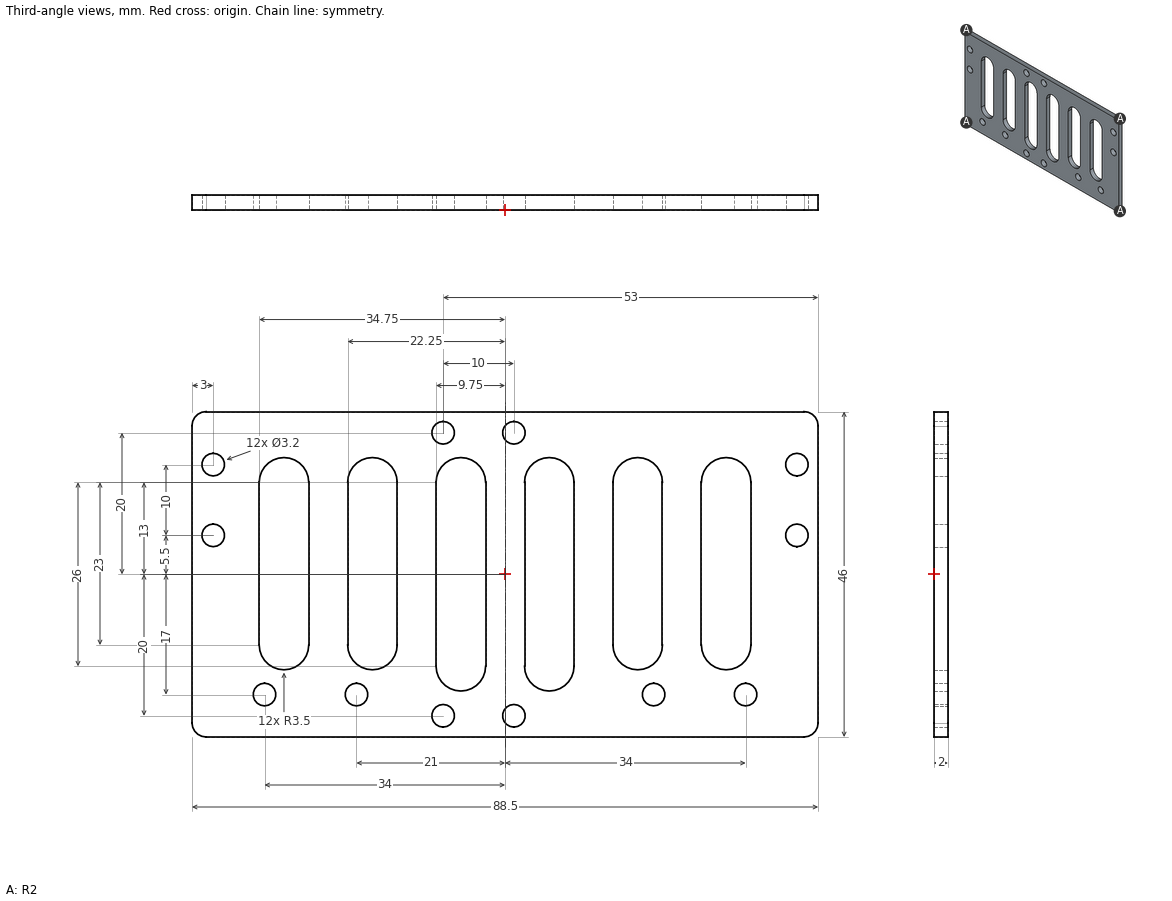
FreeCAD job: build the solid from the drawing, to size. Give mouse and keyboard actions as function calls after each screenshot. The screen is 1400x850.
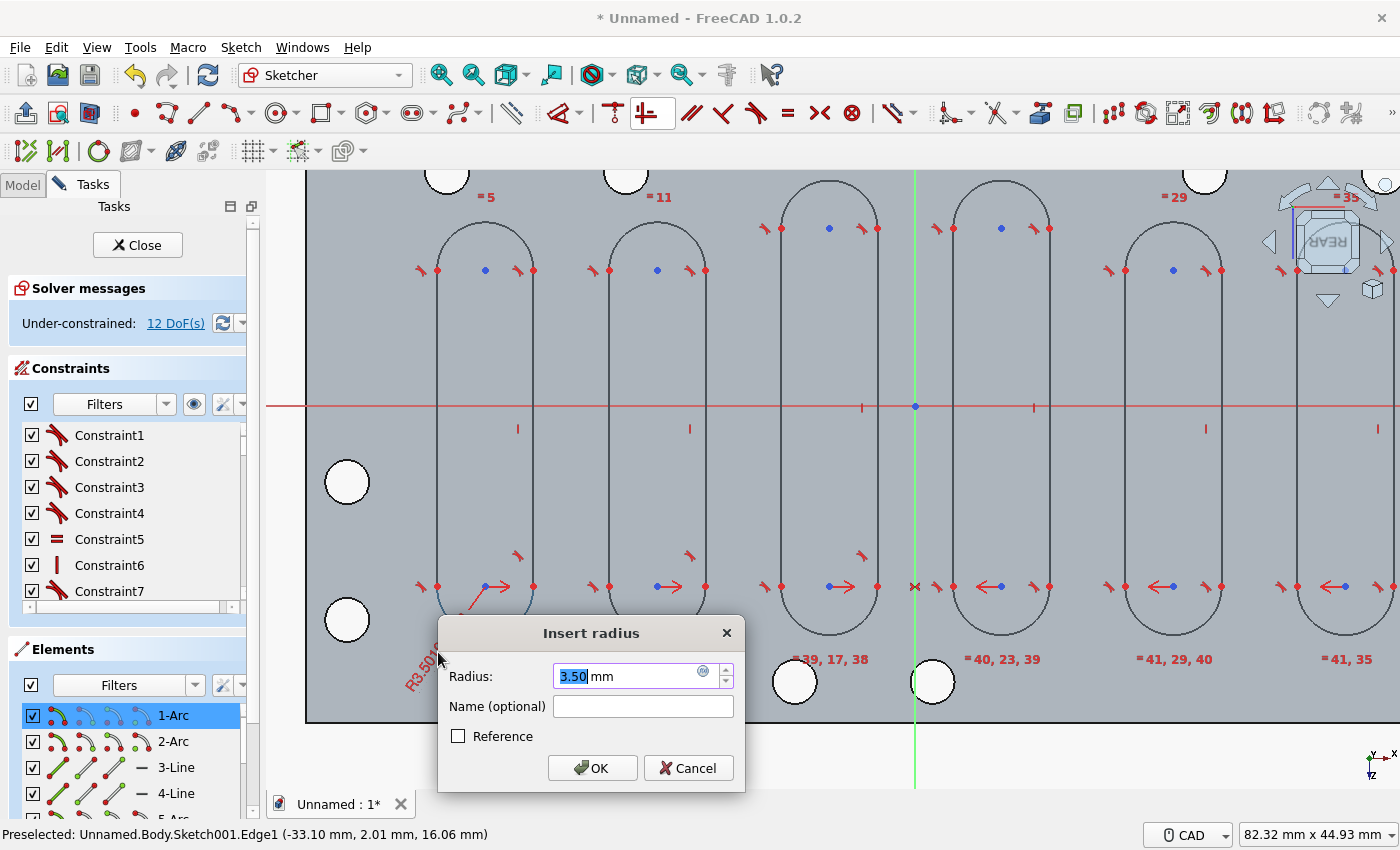
text(3.5)
key(Return)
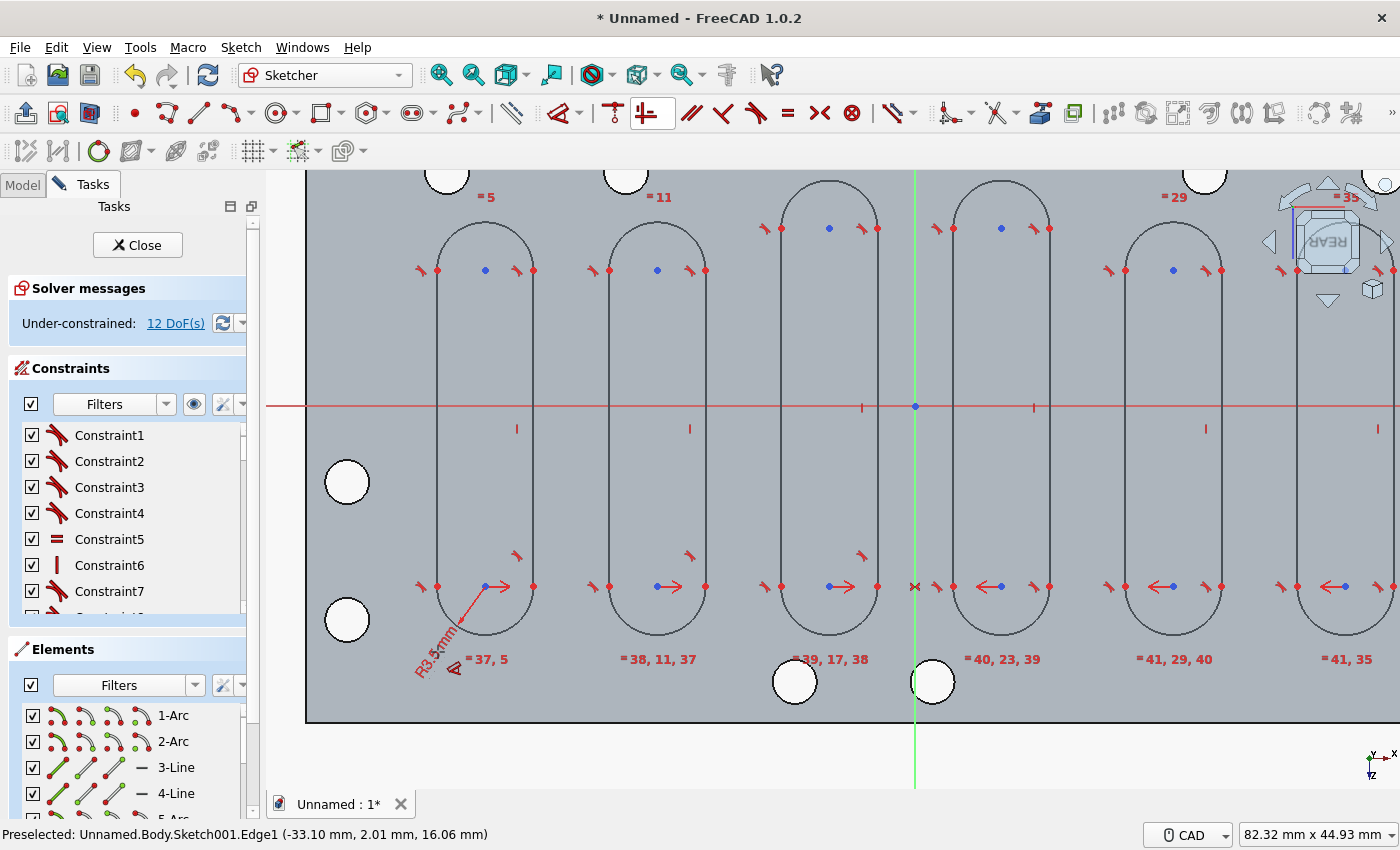
click(437, 492)
click(403, 429)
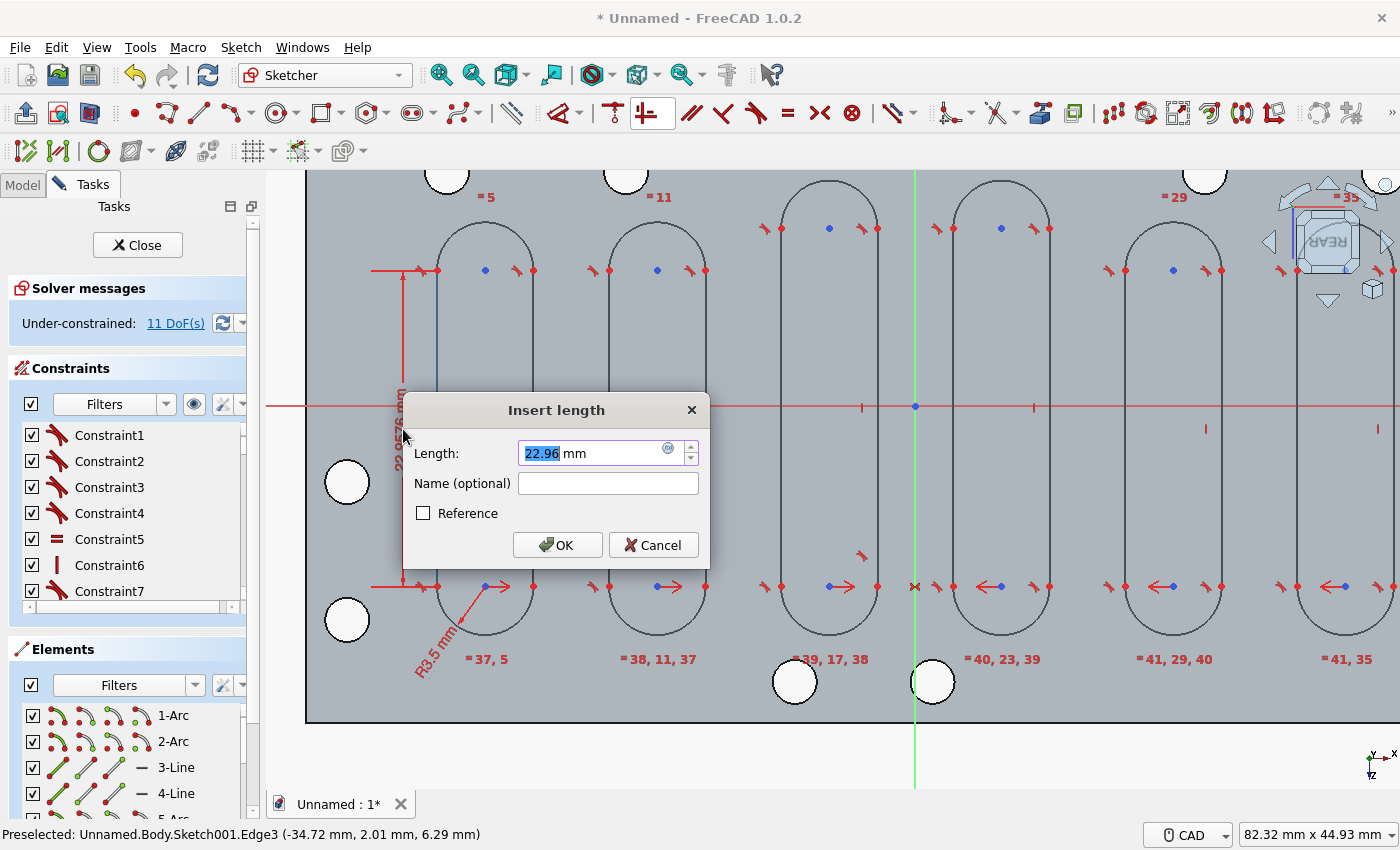
text(23)
key(Return)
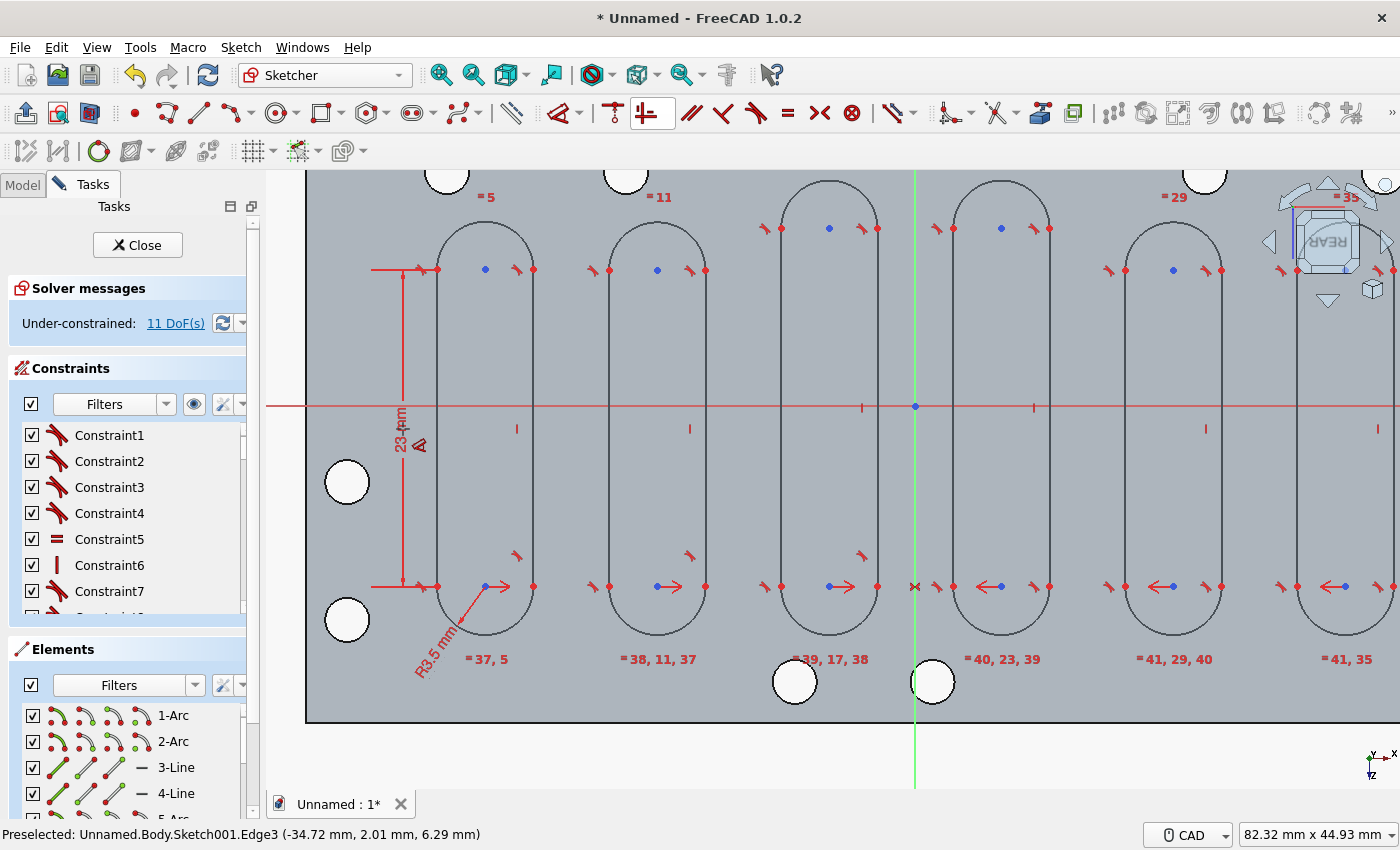
click(609, 492)
click(575, 429)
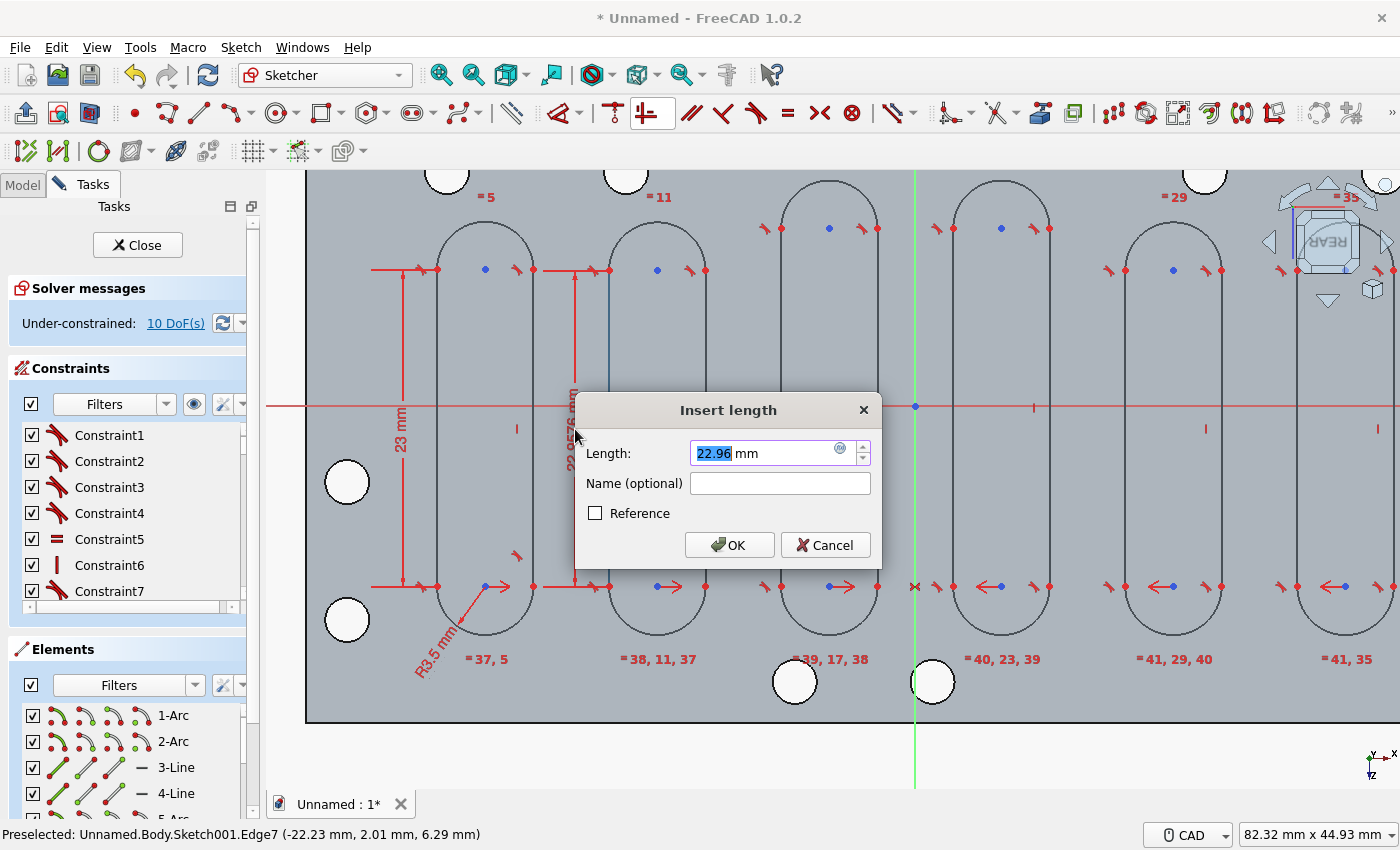
text(23)
key(Return)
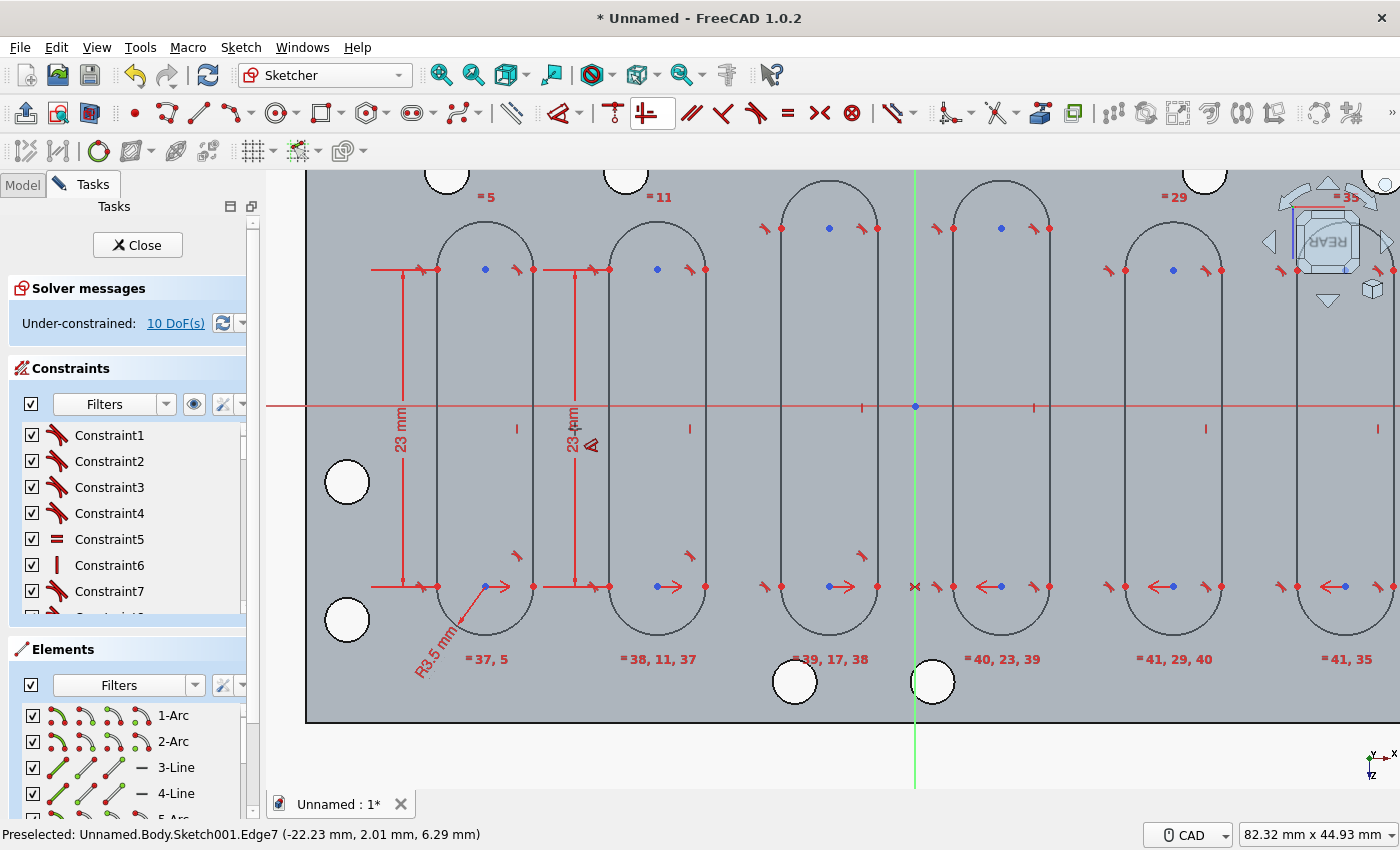
click(781, 479)
click(747, 325)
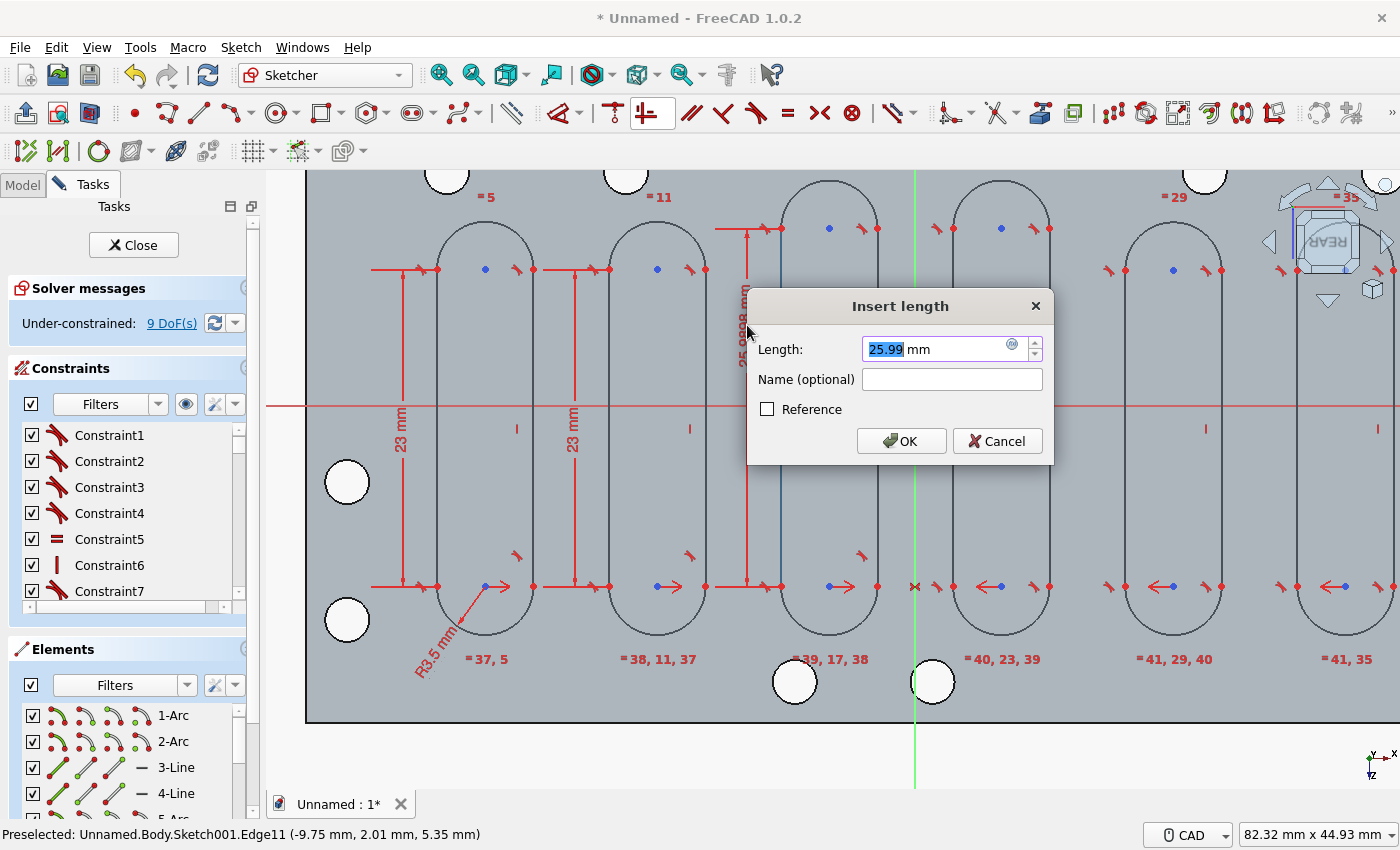
text(26)
key(Return)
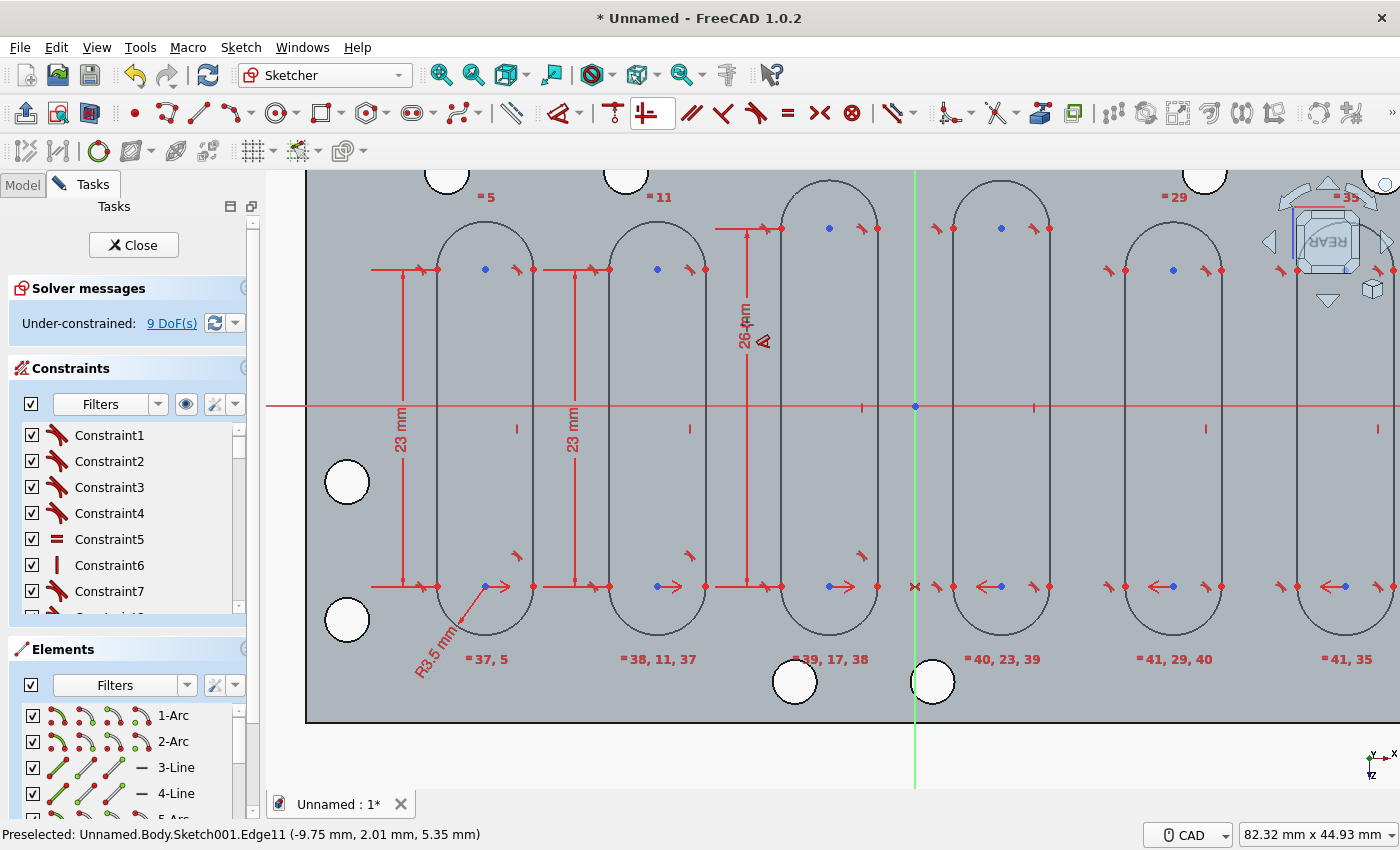
click(953, 479)
click(987, 325)